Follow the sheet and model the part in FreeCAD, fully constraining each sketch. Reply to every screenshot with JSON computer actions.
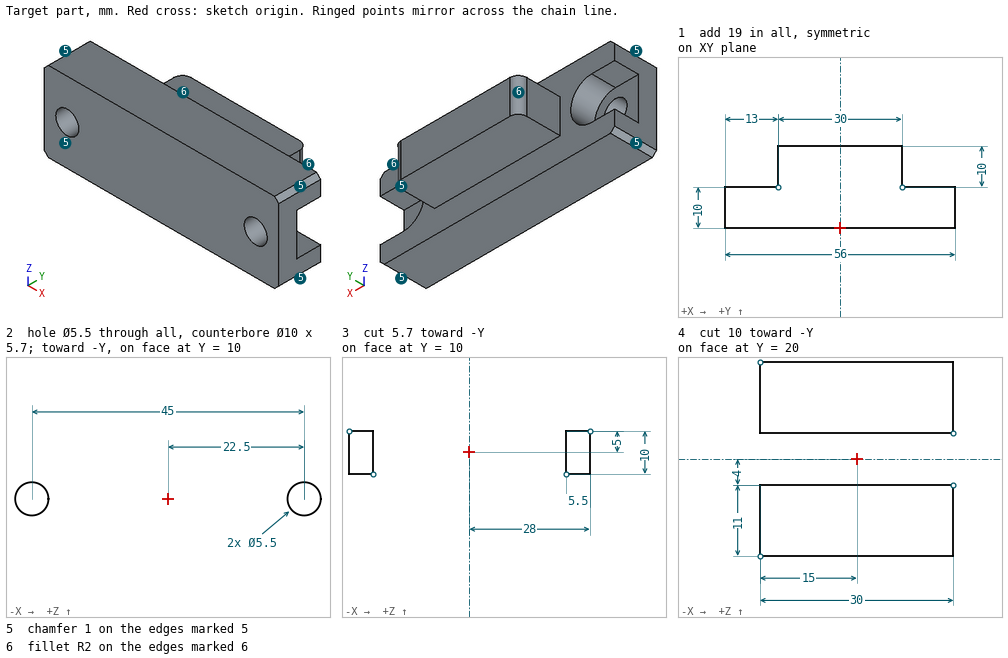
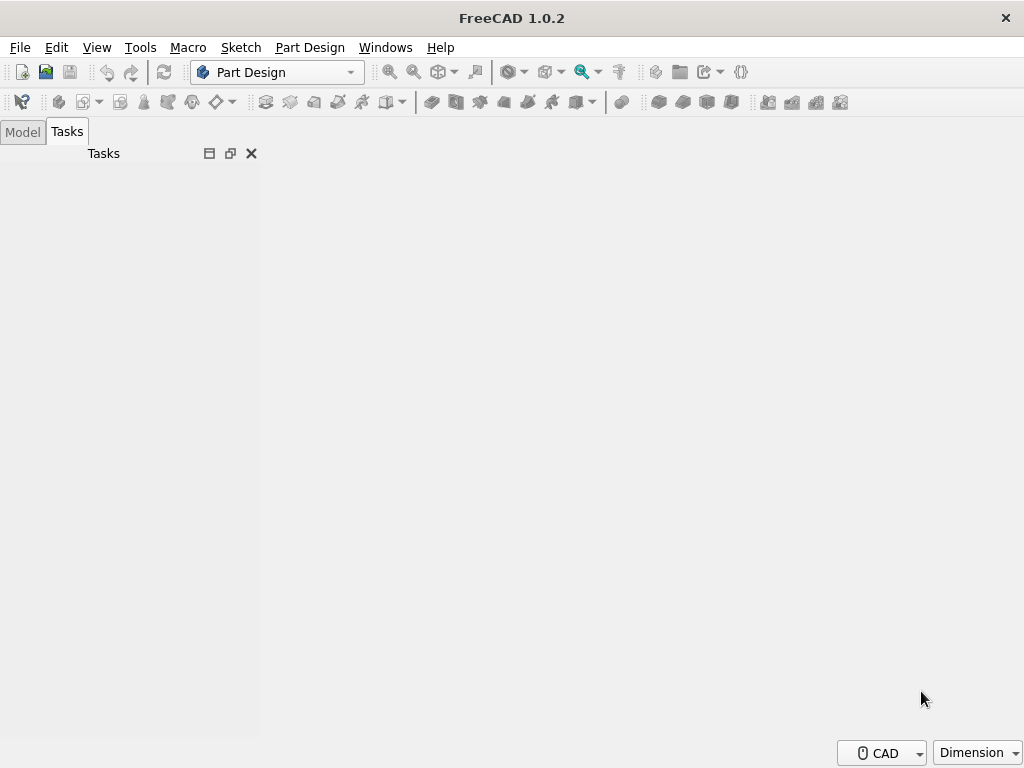
{"action": "left_click", "coordinate": [22, 72]}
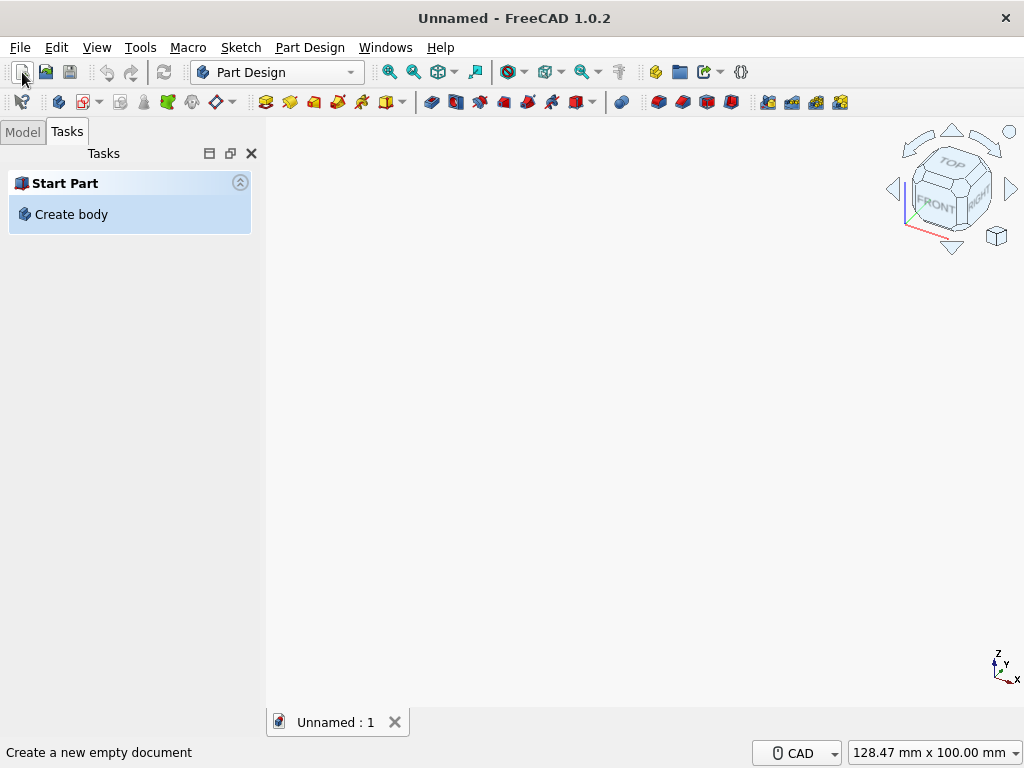
{"action": "left_click", "coordinate": [84, 102]}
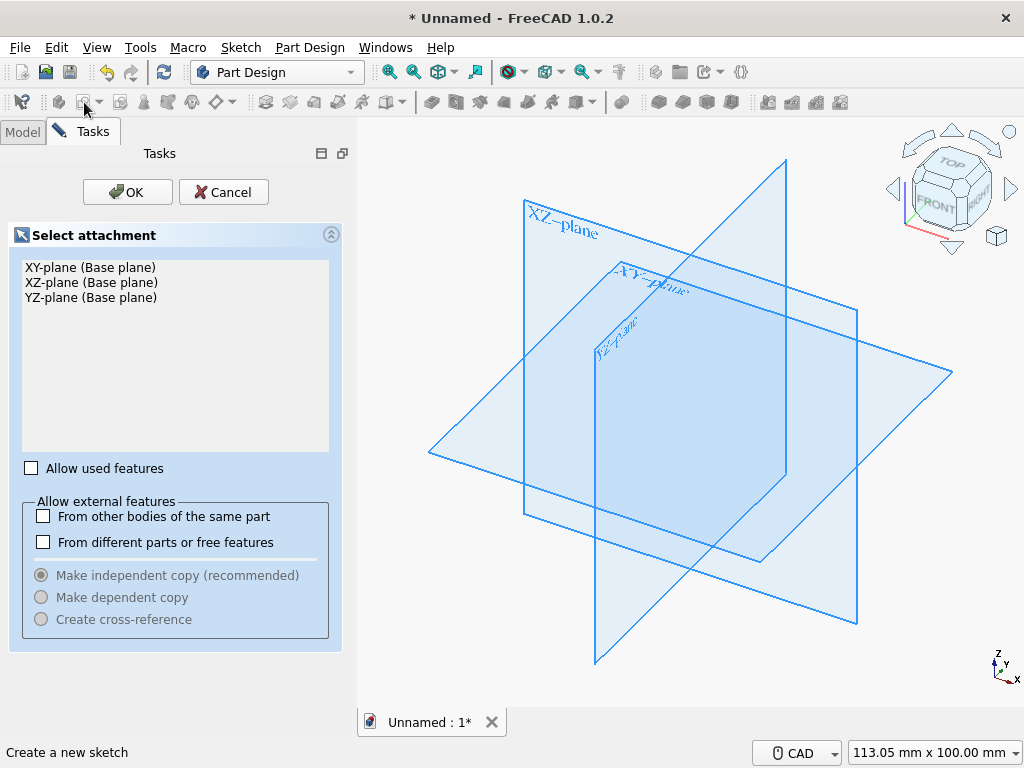
{"action": "left_click", "coordinate": [82, 268]}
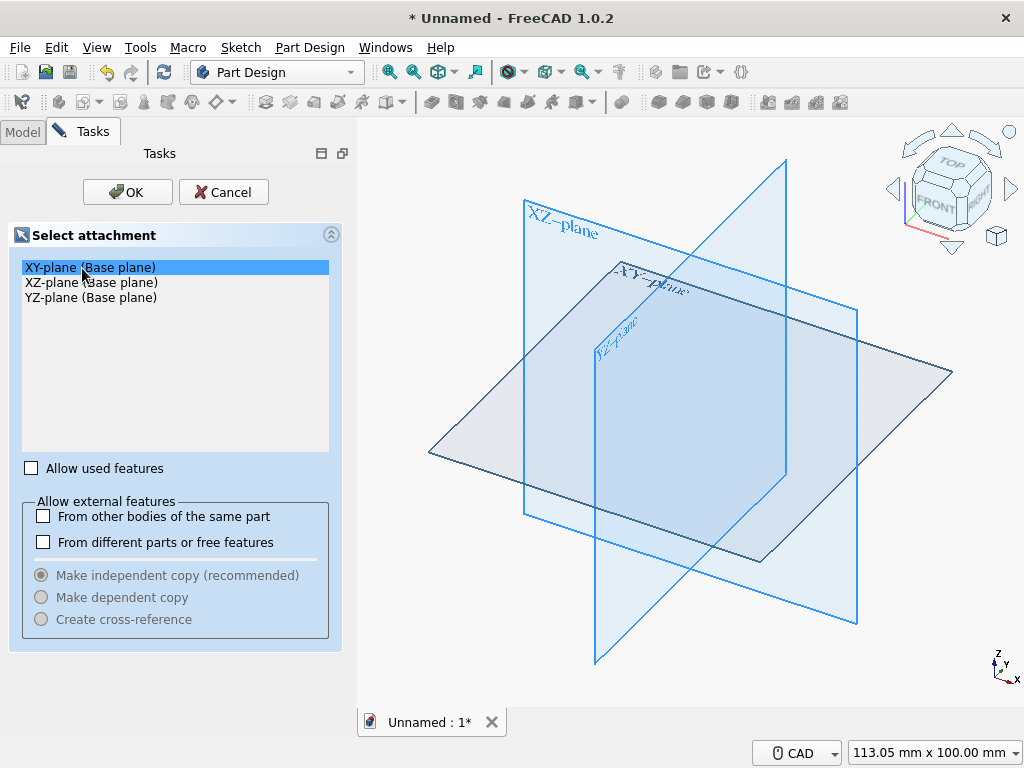
{"action": "left_click", "coordinate": [128, 192]}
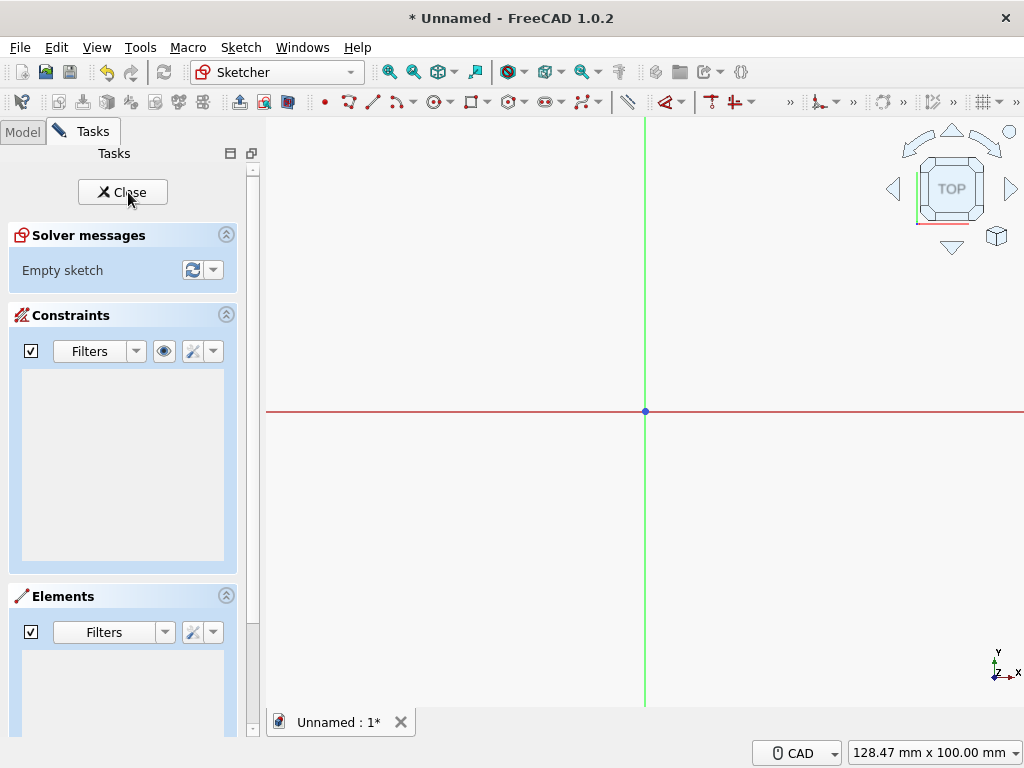
{"action": "left_click", "coordinate": [350, 102]}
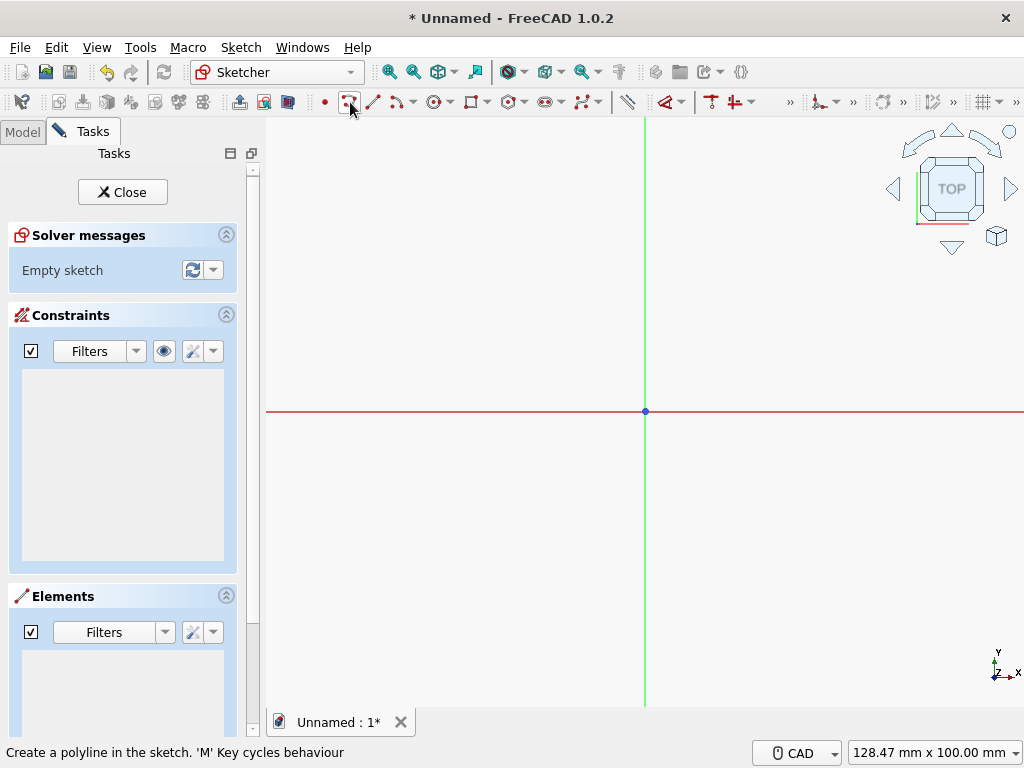
{"action": "left_click", "coordinate": [734, 353]}
{"action": "left_click", "coordinate": [734, 294]}
{"action": "left_click", "coordinate": [556, 294]}
{"action": "left_click", "coordinate": [556, 353]}
{"action": "left_click", "coordinate": [480, 353]}
{"action": "left_click", "coordinate": [480, 412]}
{"action": "left_click", "coordinate": [810, 403]}
{"action": "left_click", "coordinate": [810, 353]}
{"action": "left_click", "coordinate": [734, 354]}
{"action": "key", "text": "Escape"}
{"action": "key", "text": "Escape"}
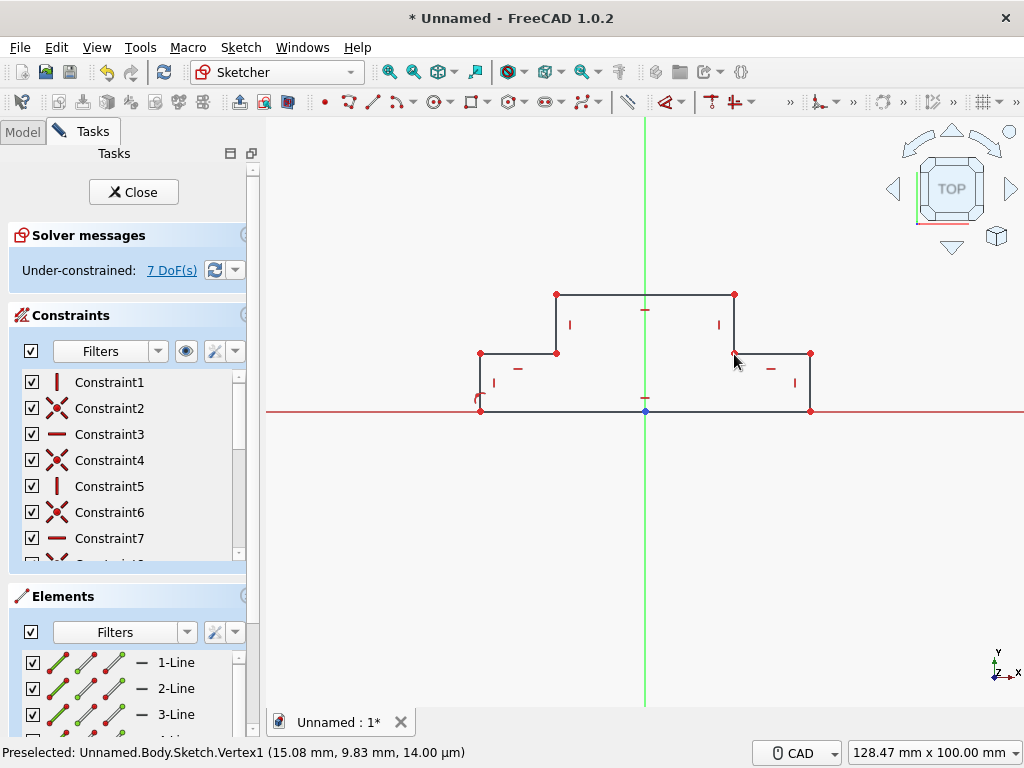
{"action": "left_click", "coordinate": [734, 354]}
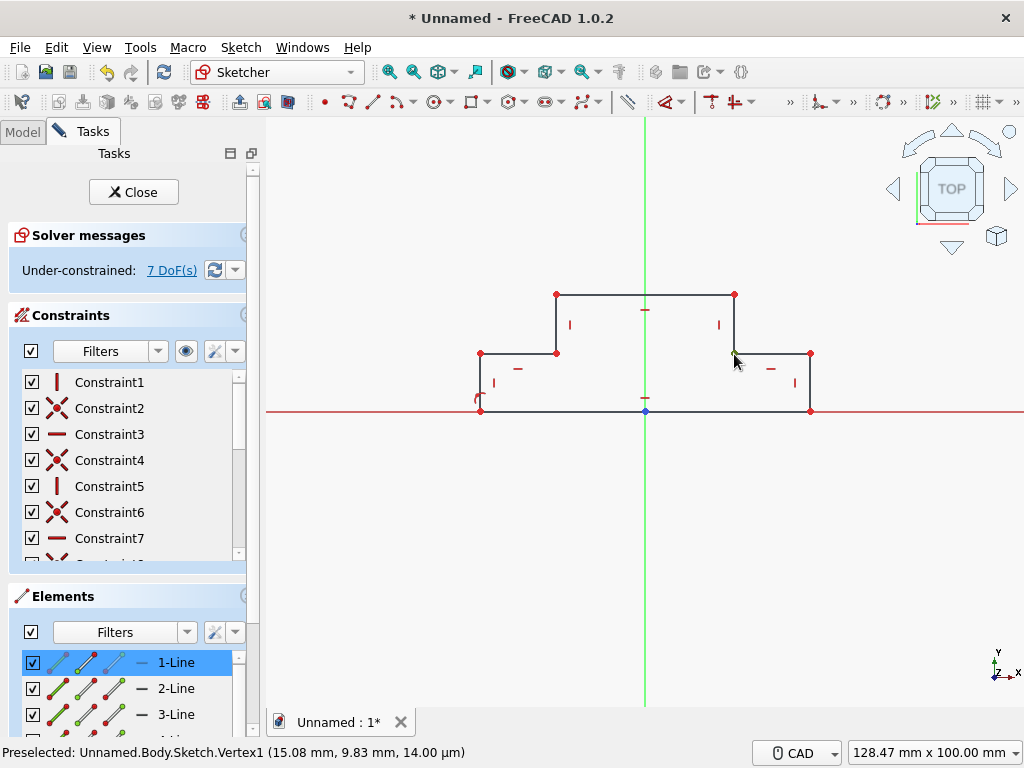
{"action": "left_click", "coordinate": [556, 354]}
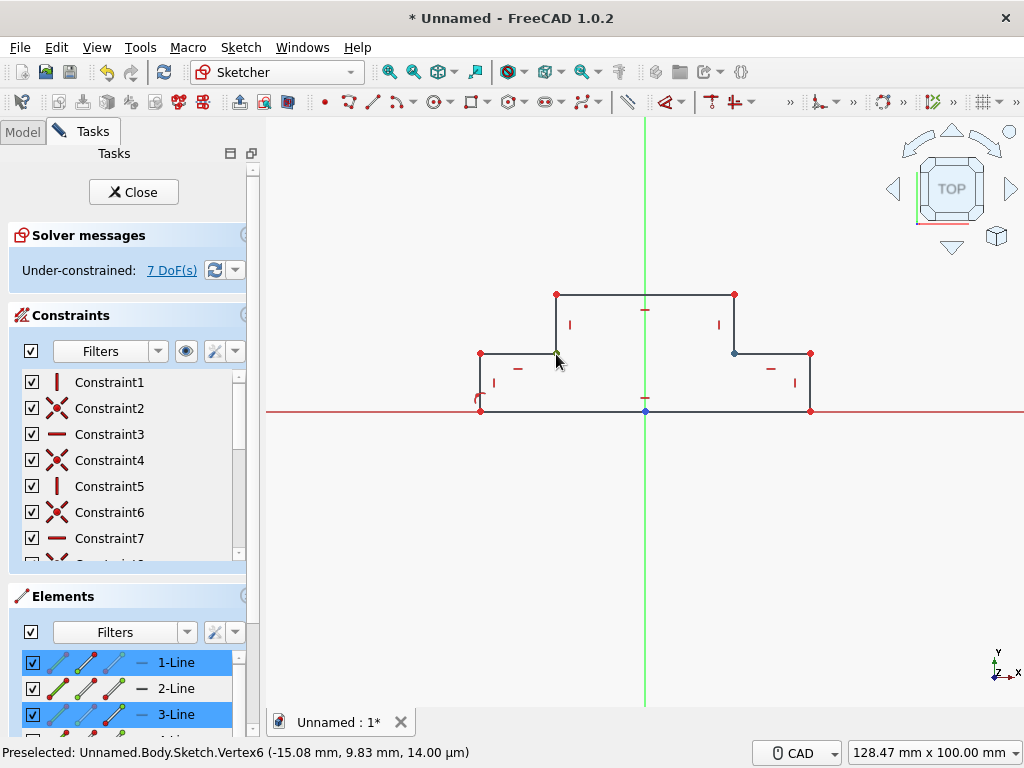
{"action": "left_click", "coordinate": [645, 641]}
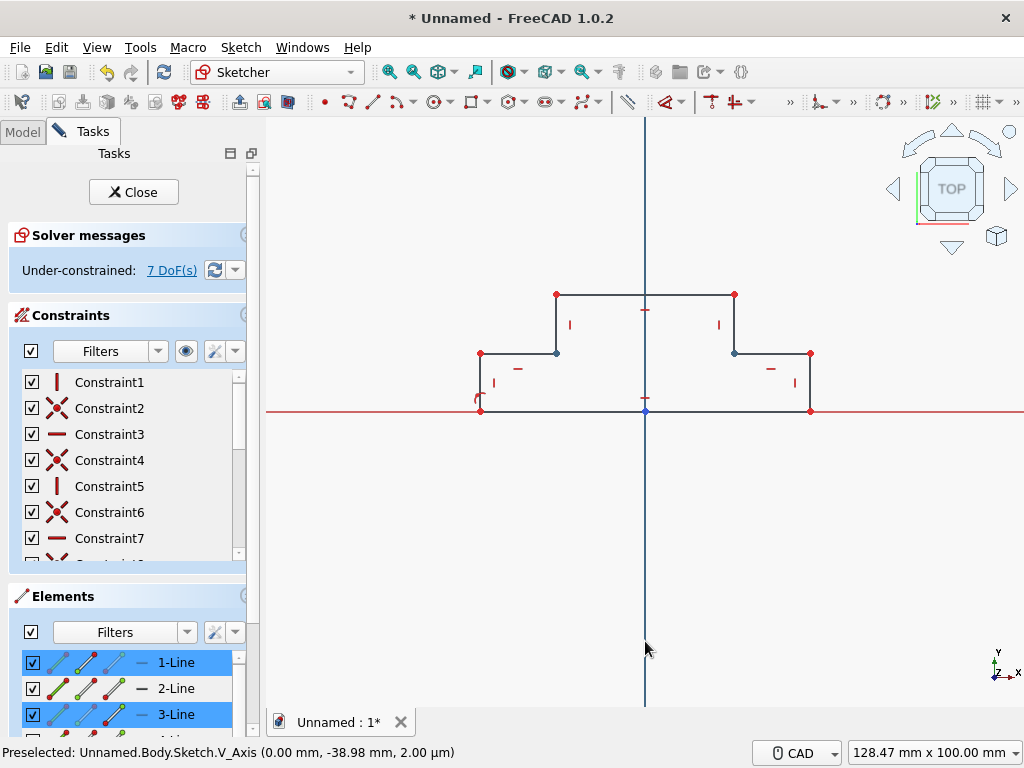
{"action": "key", "text": "s"}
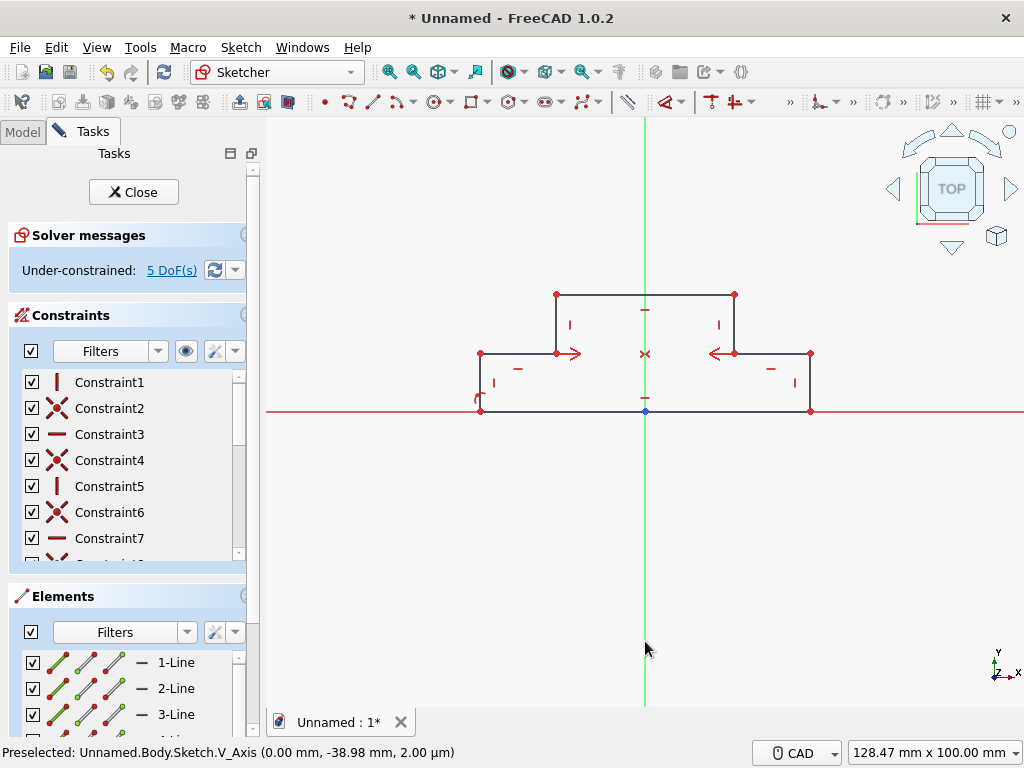
{"action": "left_click", "coordinate": [666, 102]}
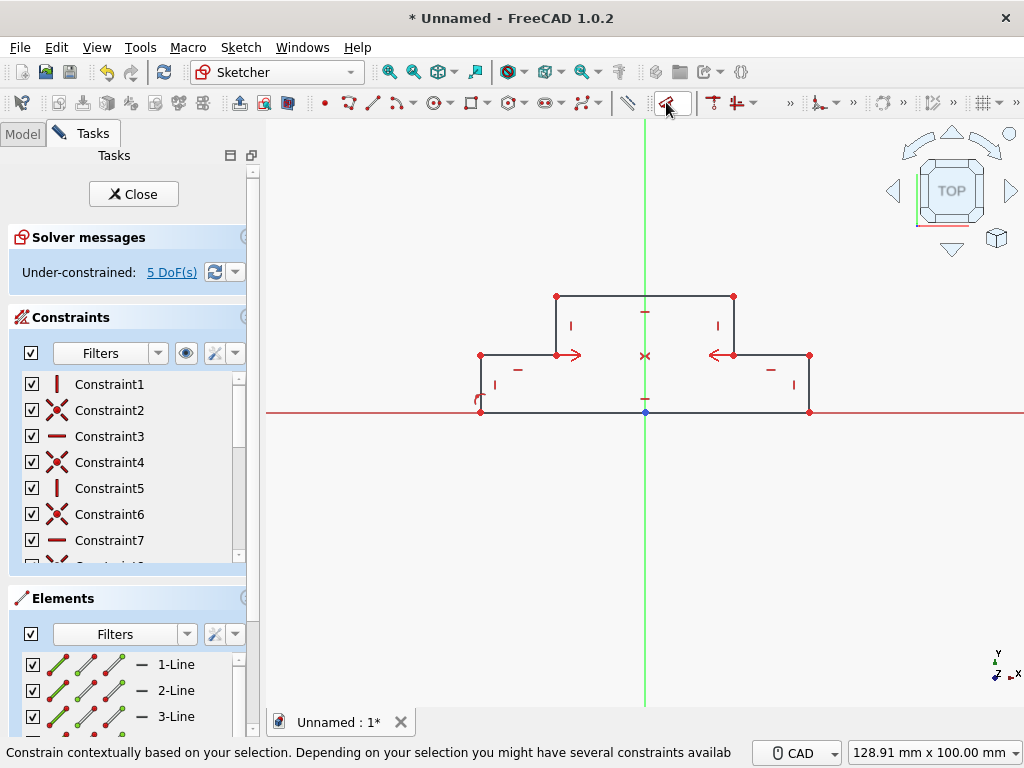
{"action": "left_click", "coordinate": [734, 338]}
{"action": "left_click", "coordinate": [768, 326]}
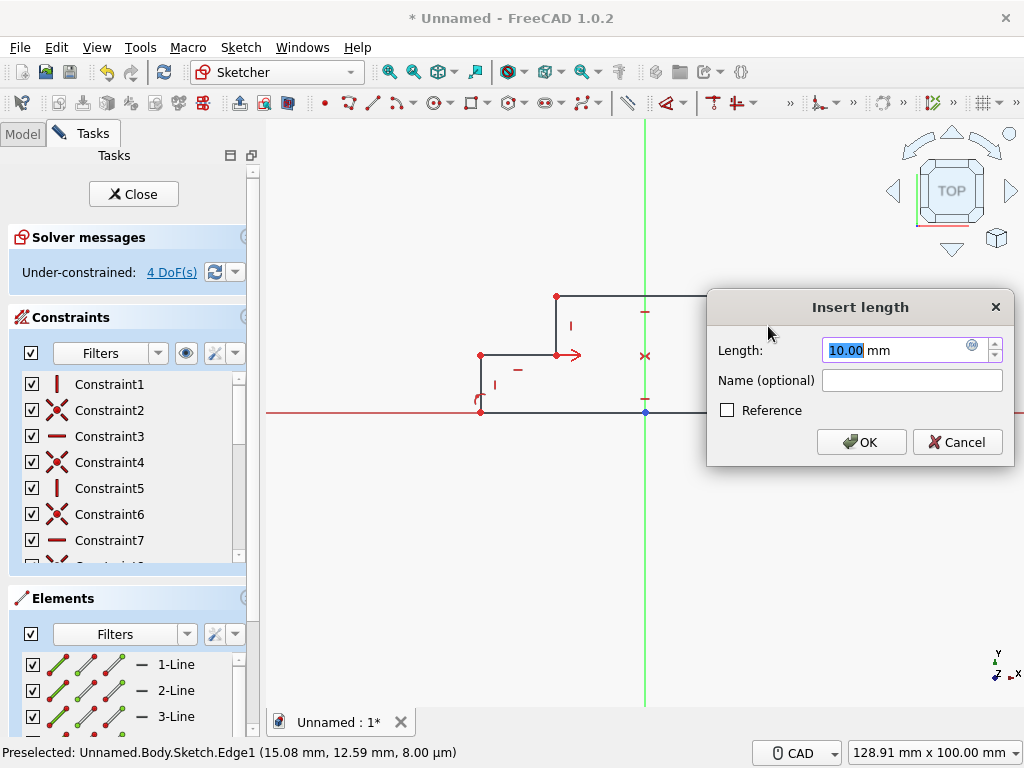
{"action": "type", "text": "10"}
{"action": "key", "text": "Return"}